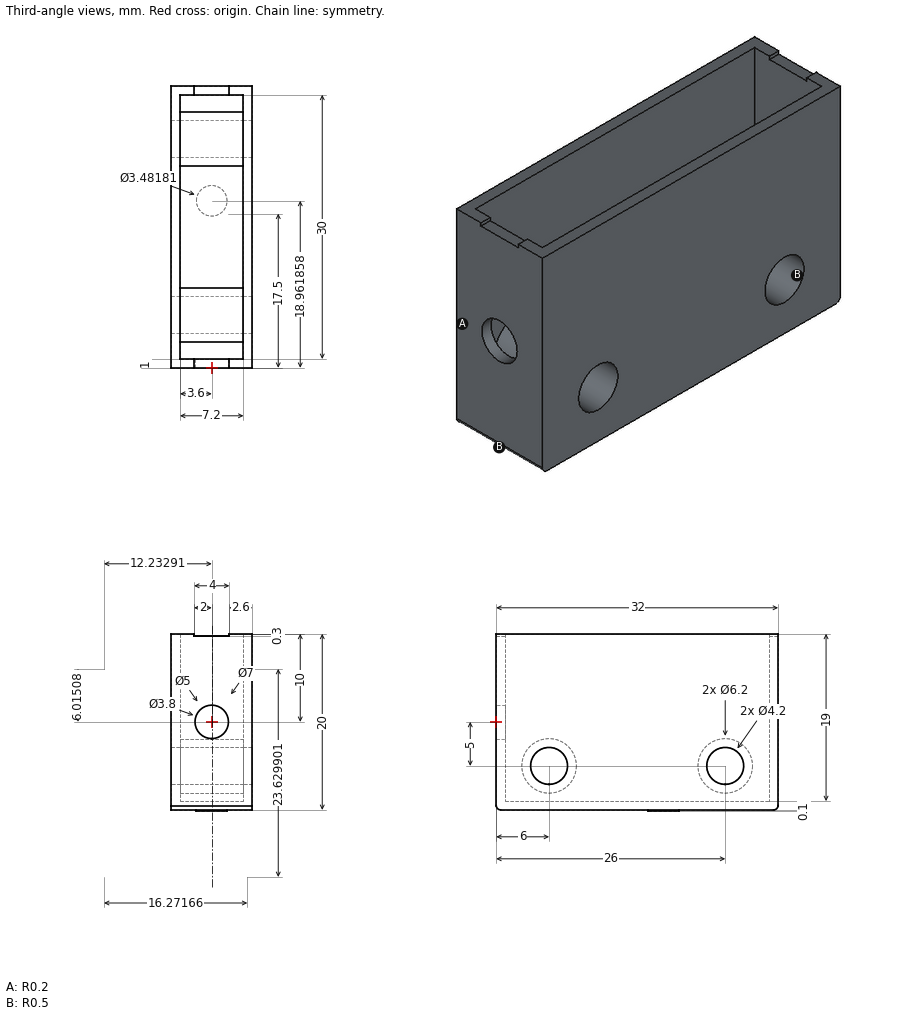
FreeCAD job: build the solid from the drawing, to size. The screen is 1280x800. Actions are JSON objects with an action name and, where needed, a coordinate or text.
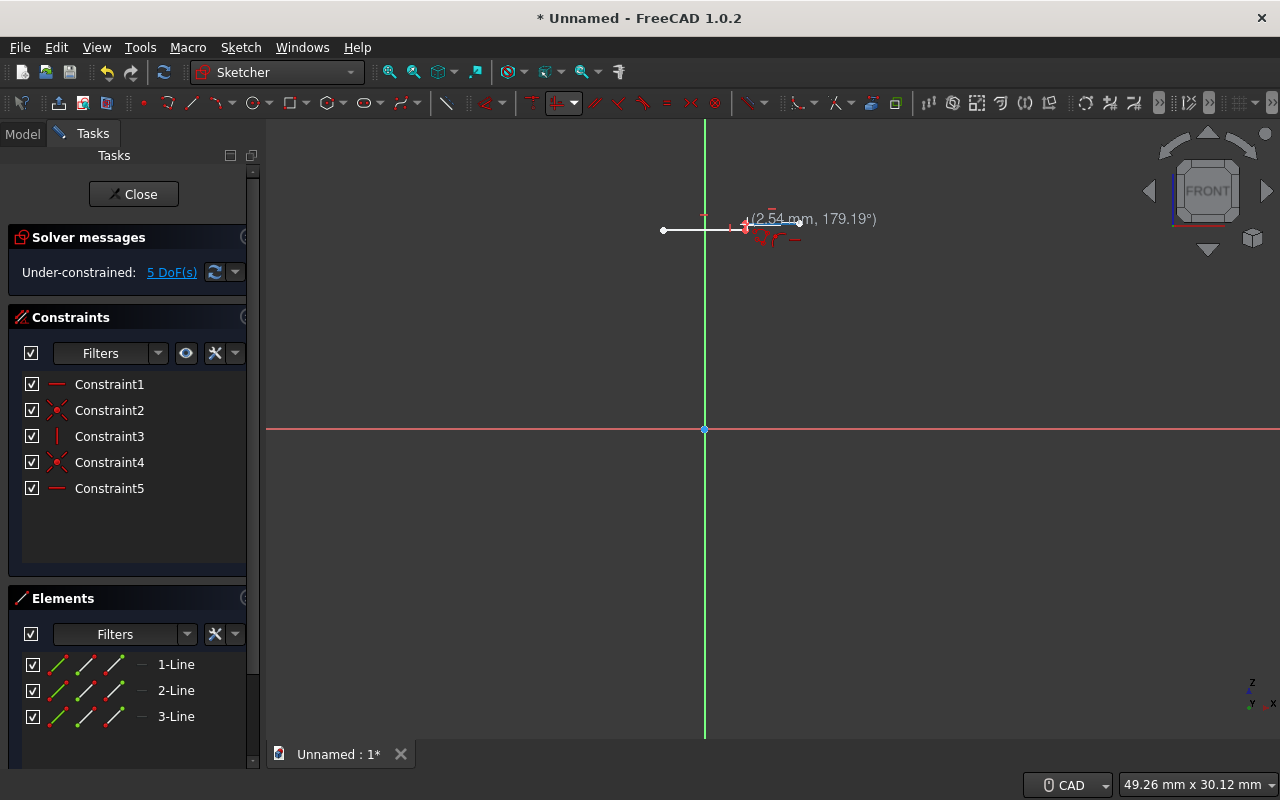
{"action": "left_click", "coordinate": [800, 635]}
{"action": "left_click", "coordinate": [610, 635]}
{"action": "left_click", "coordinate": [610, 223]}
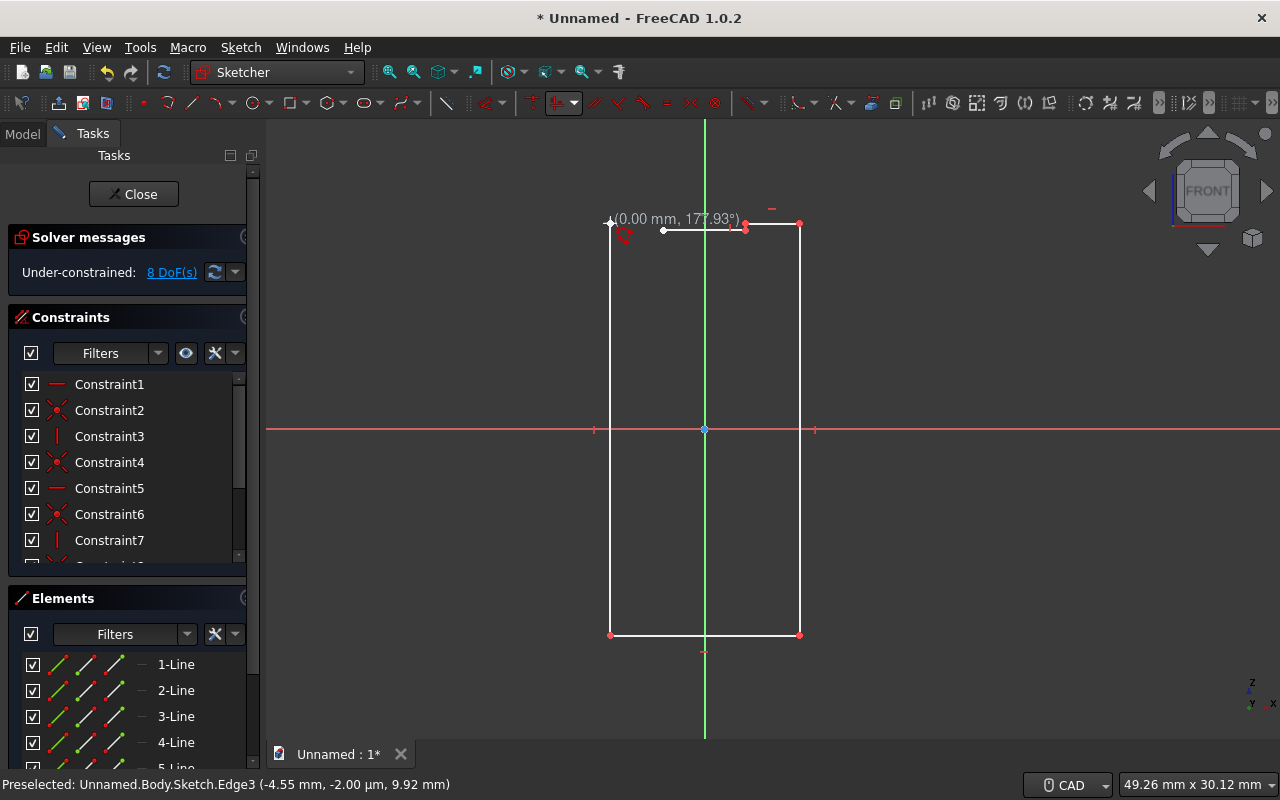
{"action": "scroll", "coordinate": [664, 223], "scroll_direction": "up", "scroll_amount": 5}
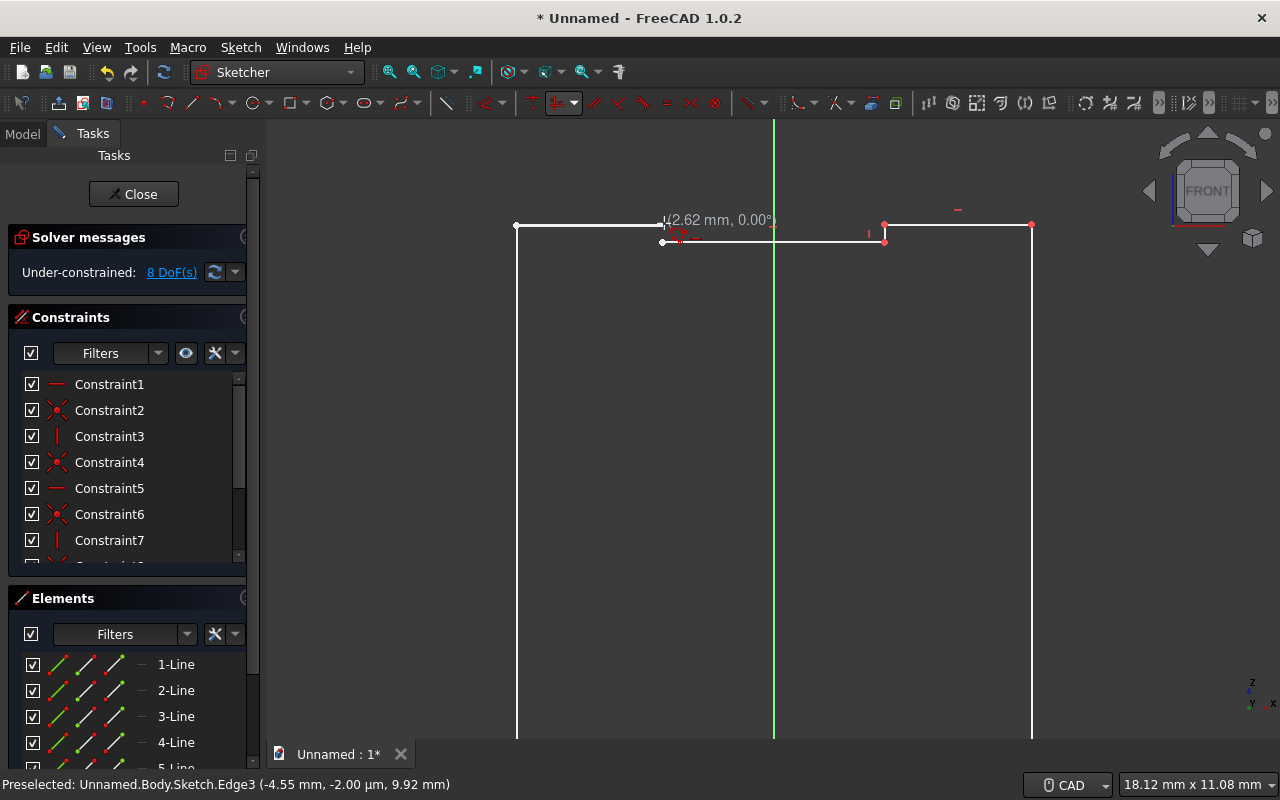
{"action": "left_click", "coordinate": [662, 223]}
{"action": "left_click", "coordinate": [662, 242]}
{"action": "key", "text": "Escape"}
{"action": "key", "text": "Escape"}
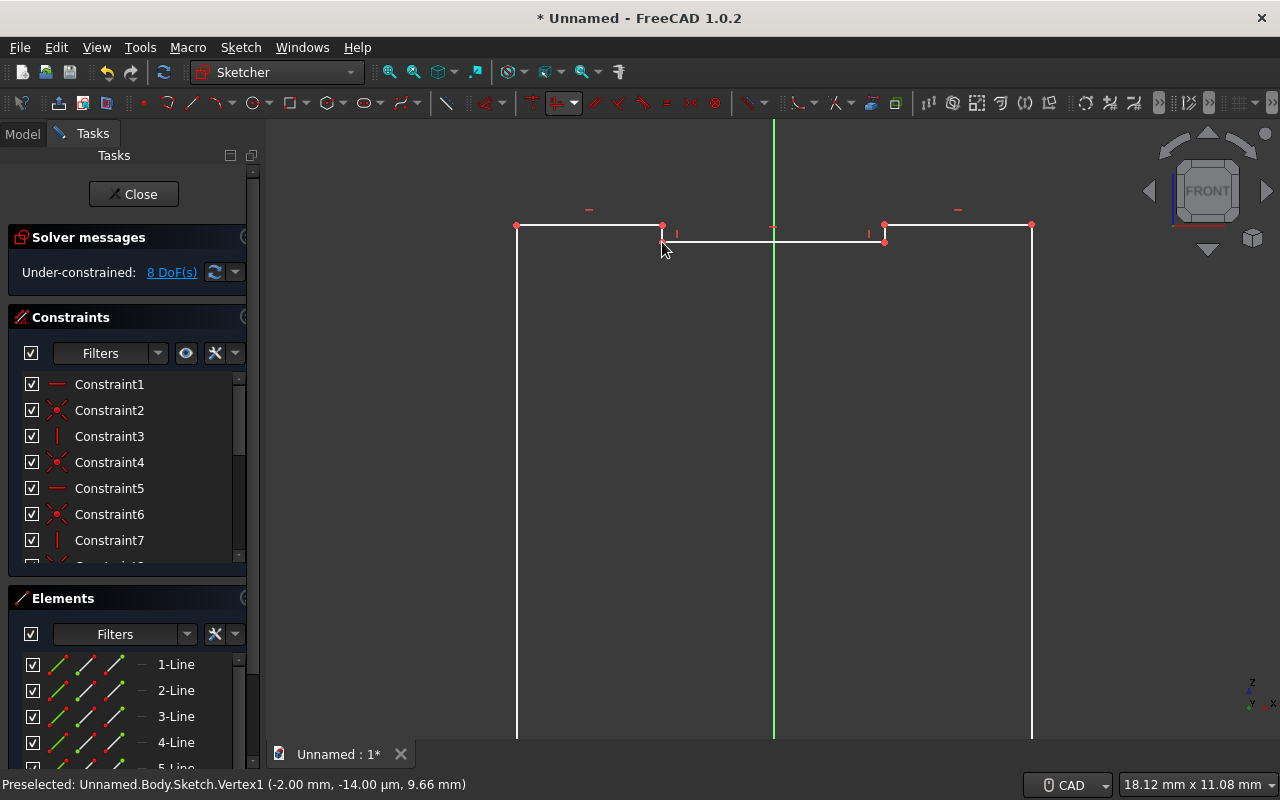
{"action": "left_click", "coordinate": [1032, 225]}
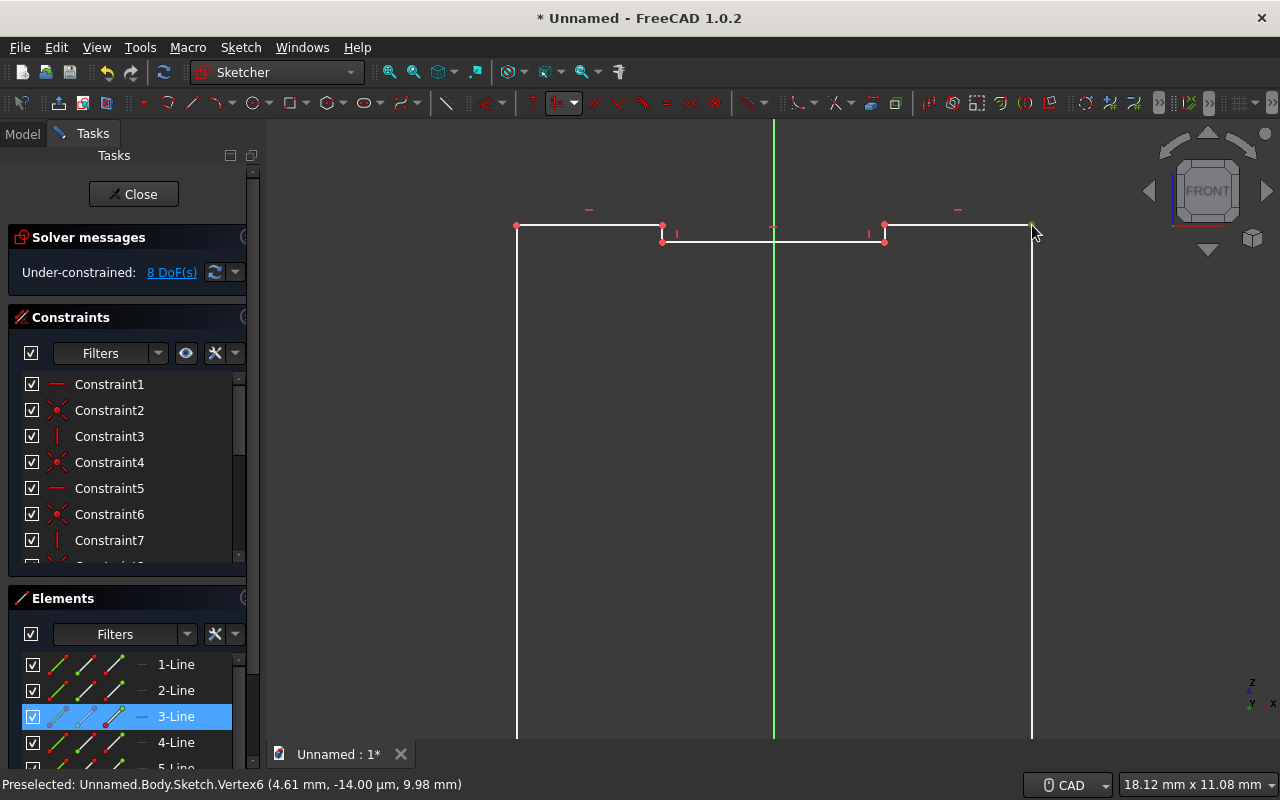
{"action": "left_click", "coordinate": [517, 225]}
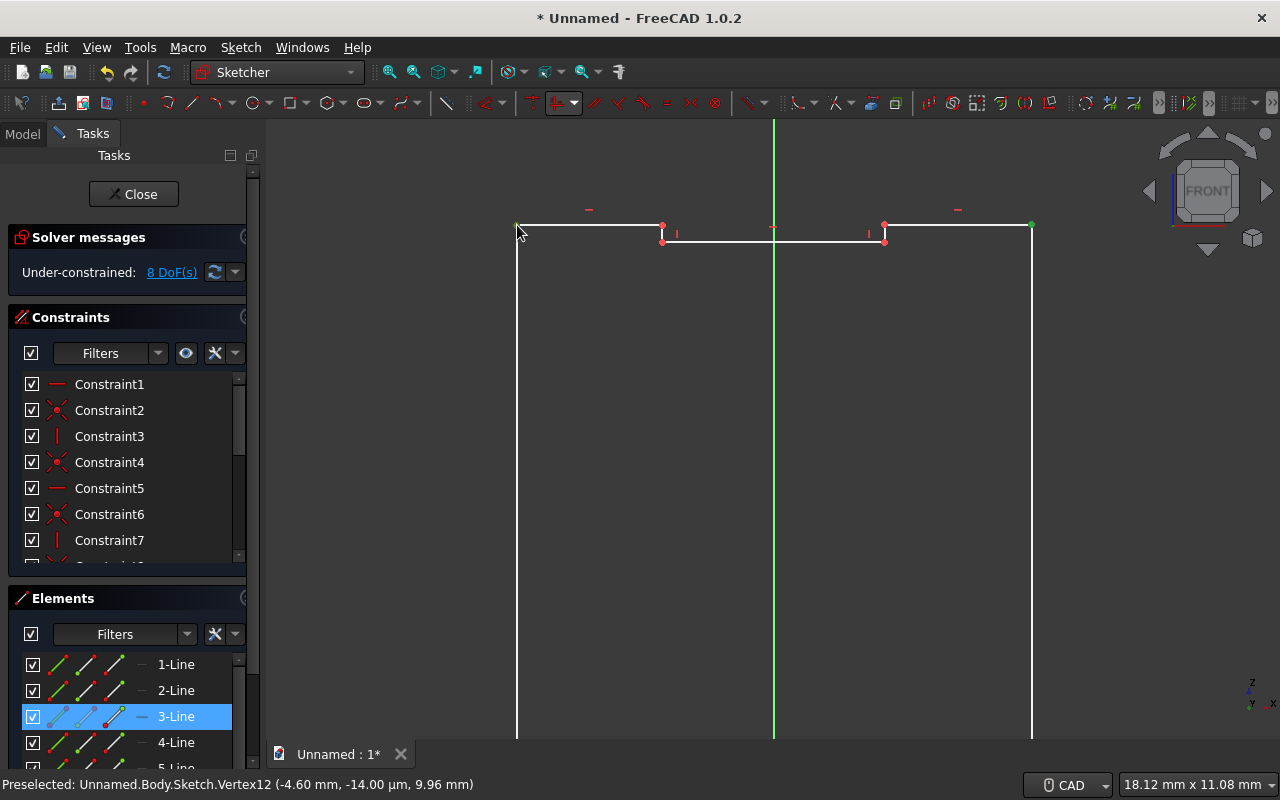
{"action": "left_click", "coordinate": [774, 671]}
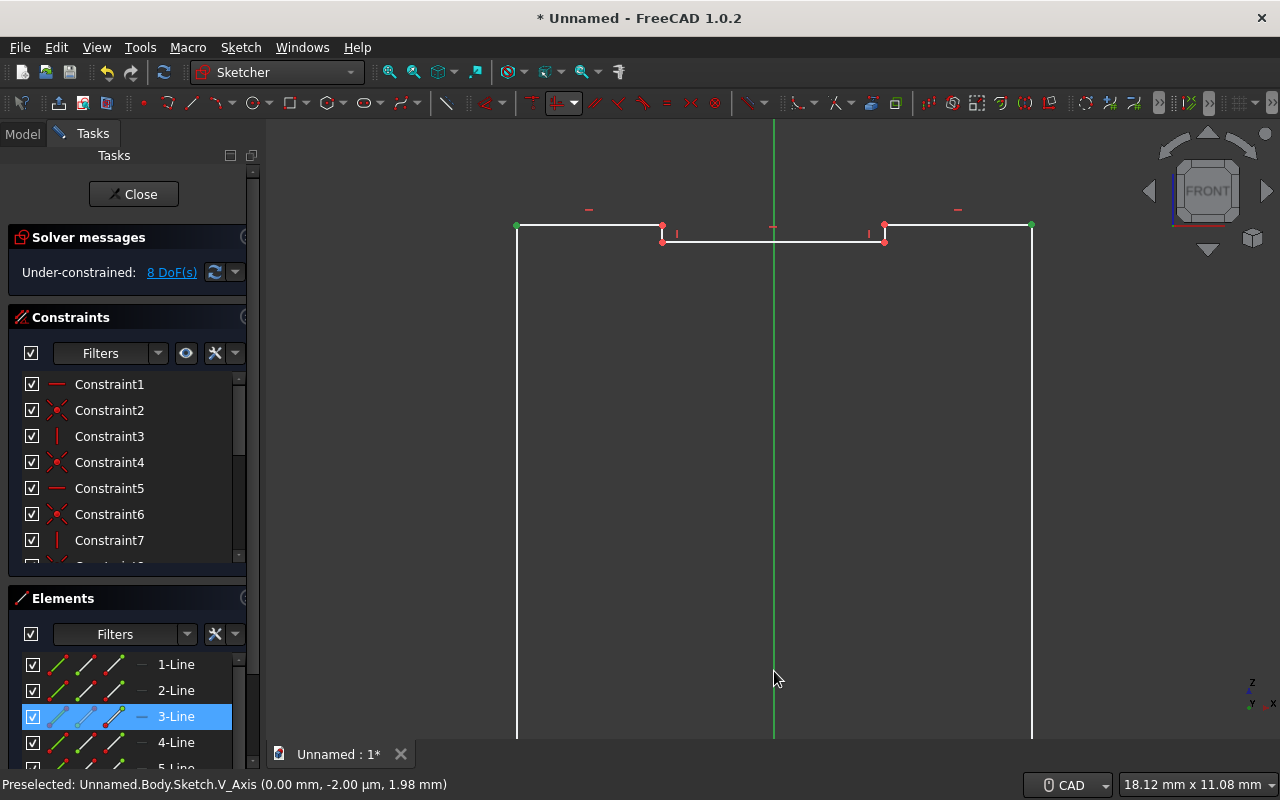
{"action": "left_click", "coordinate": [692, 104]}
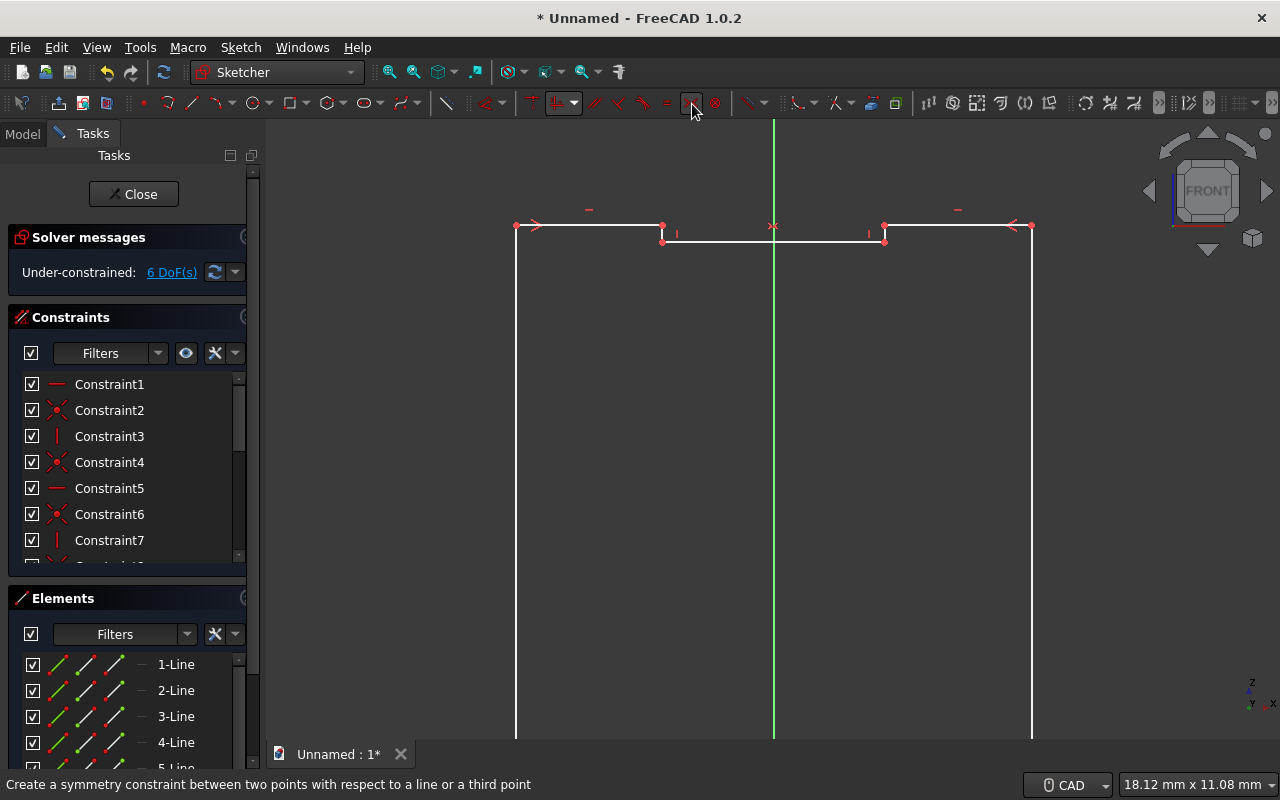
{"action": "left_click", "coordinate": [729, 242]}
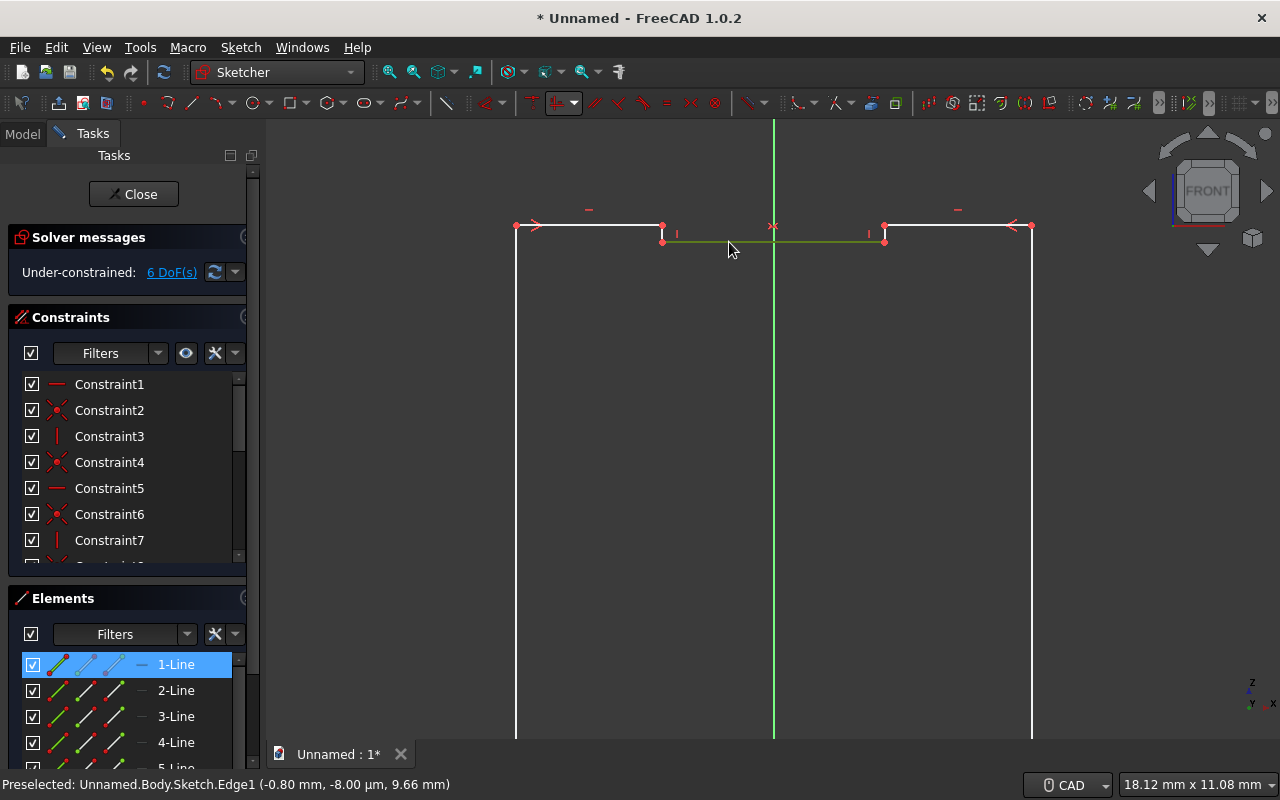
{"action": "left_click", "coordinate": [504, 104]}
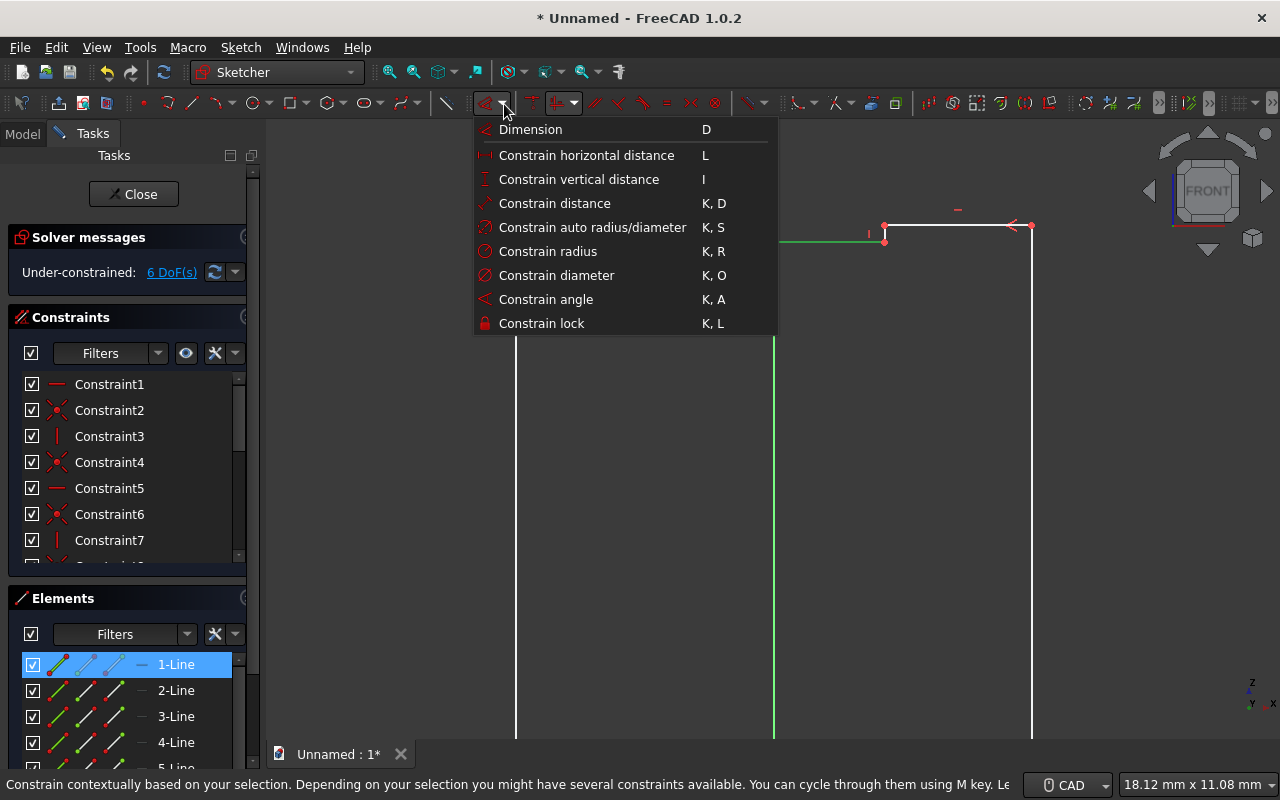
{"action": "left_click", "coordinate": [626, 155]}